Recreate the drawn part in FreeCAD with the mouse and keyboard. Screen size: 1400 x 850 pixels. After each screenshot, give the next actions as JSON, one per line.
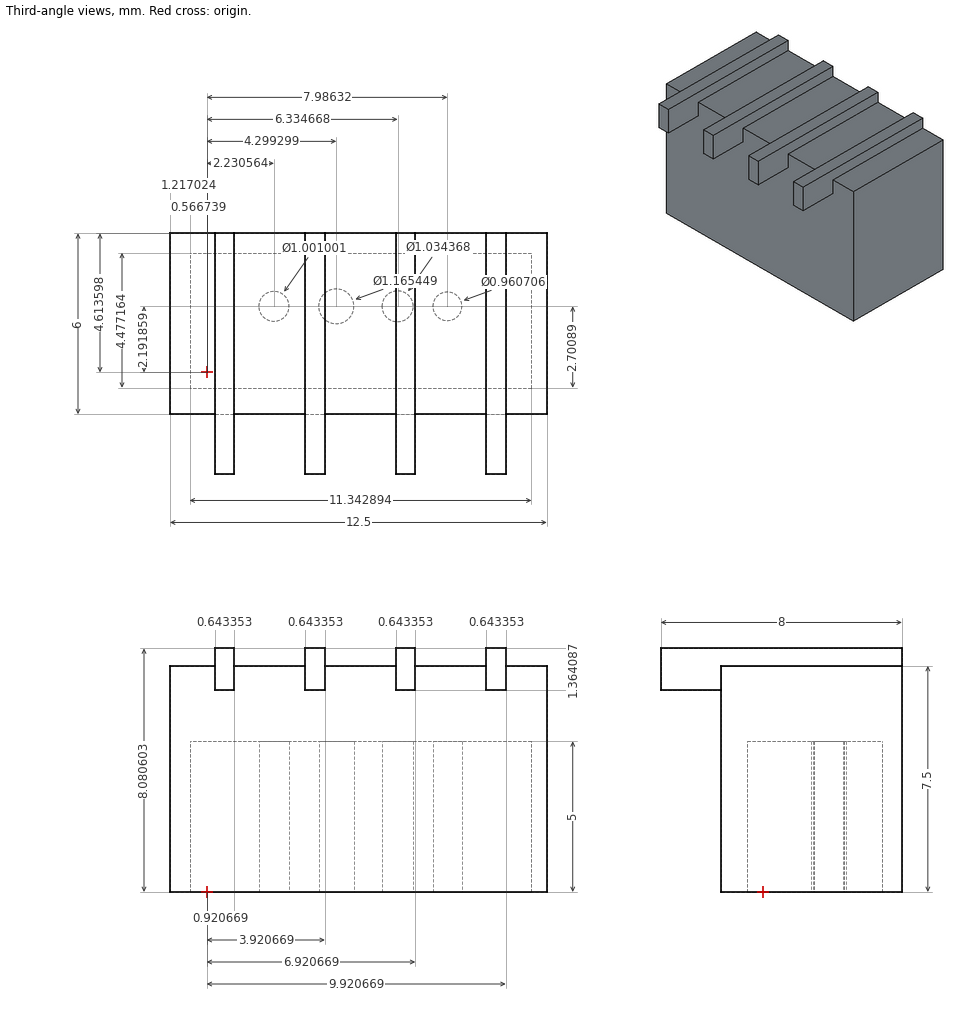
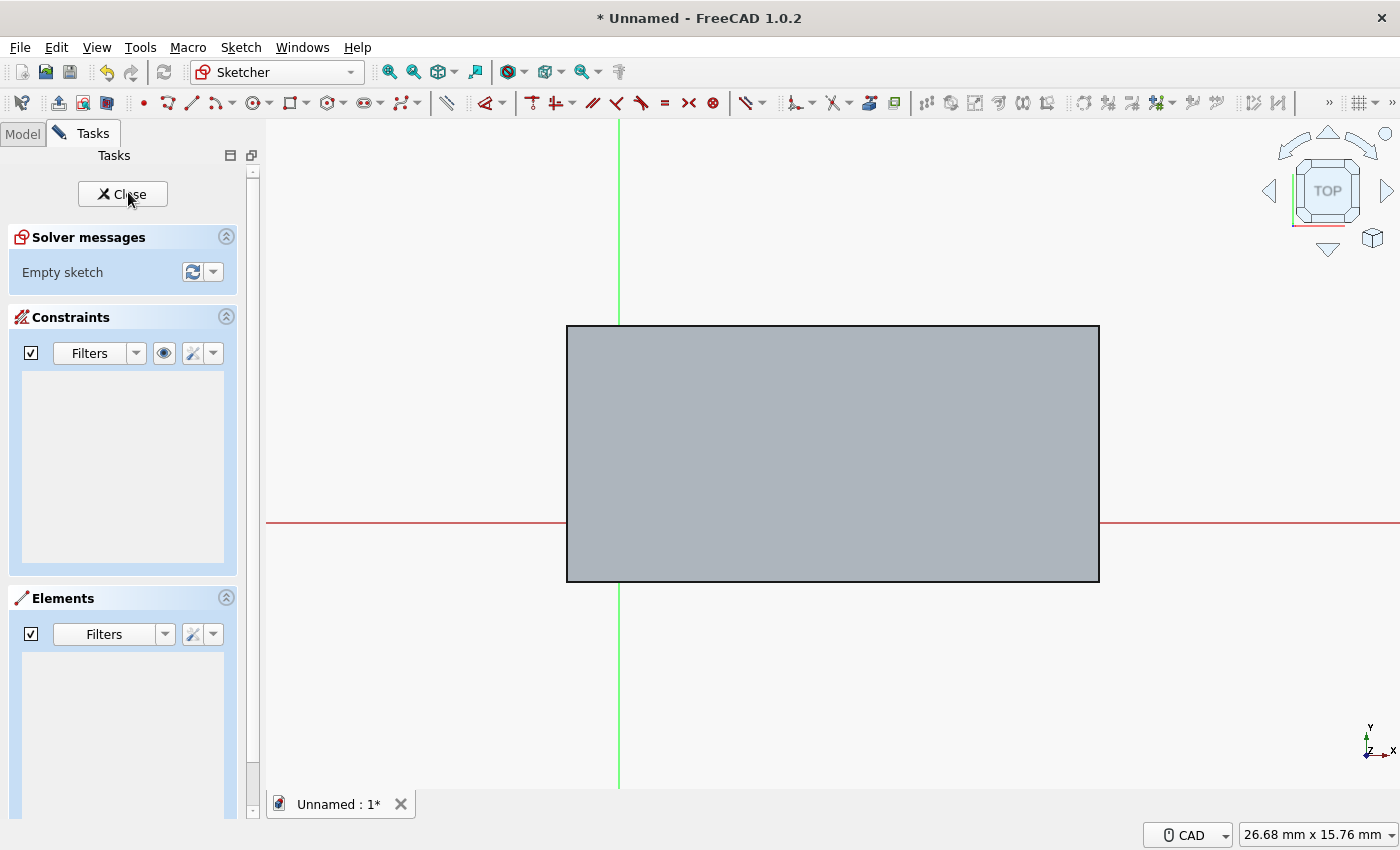
{"action": "key", "text": "q s"}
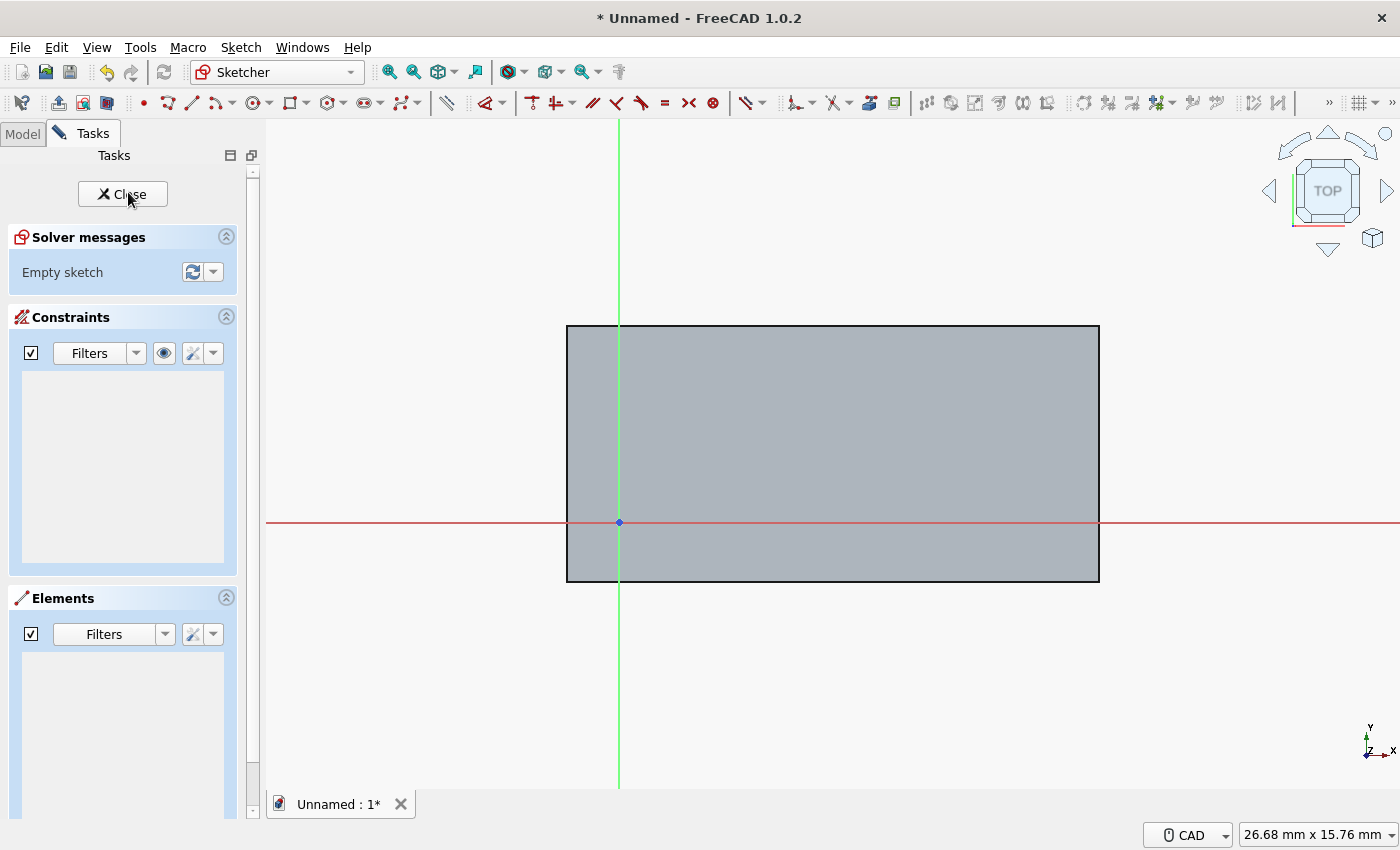
{"action": "scroll", "coordinate": [982, 439], "scroll_direction": "up", "scroll_amount": 2}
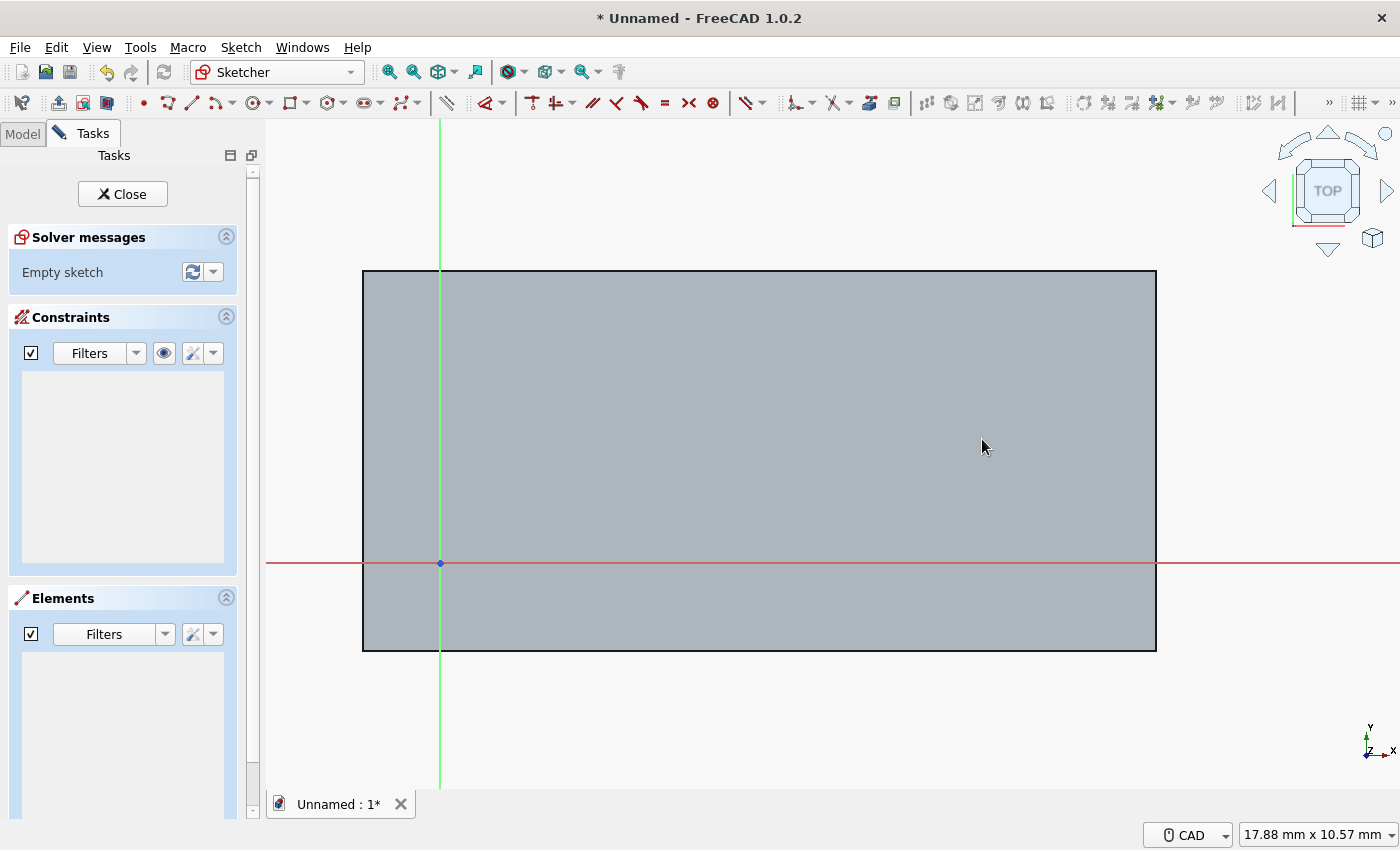
{"action": "left_click", "coordinate": [290, 104]}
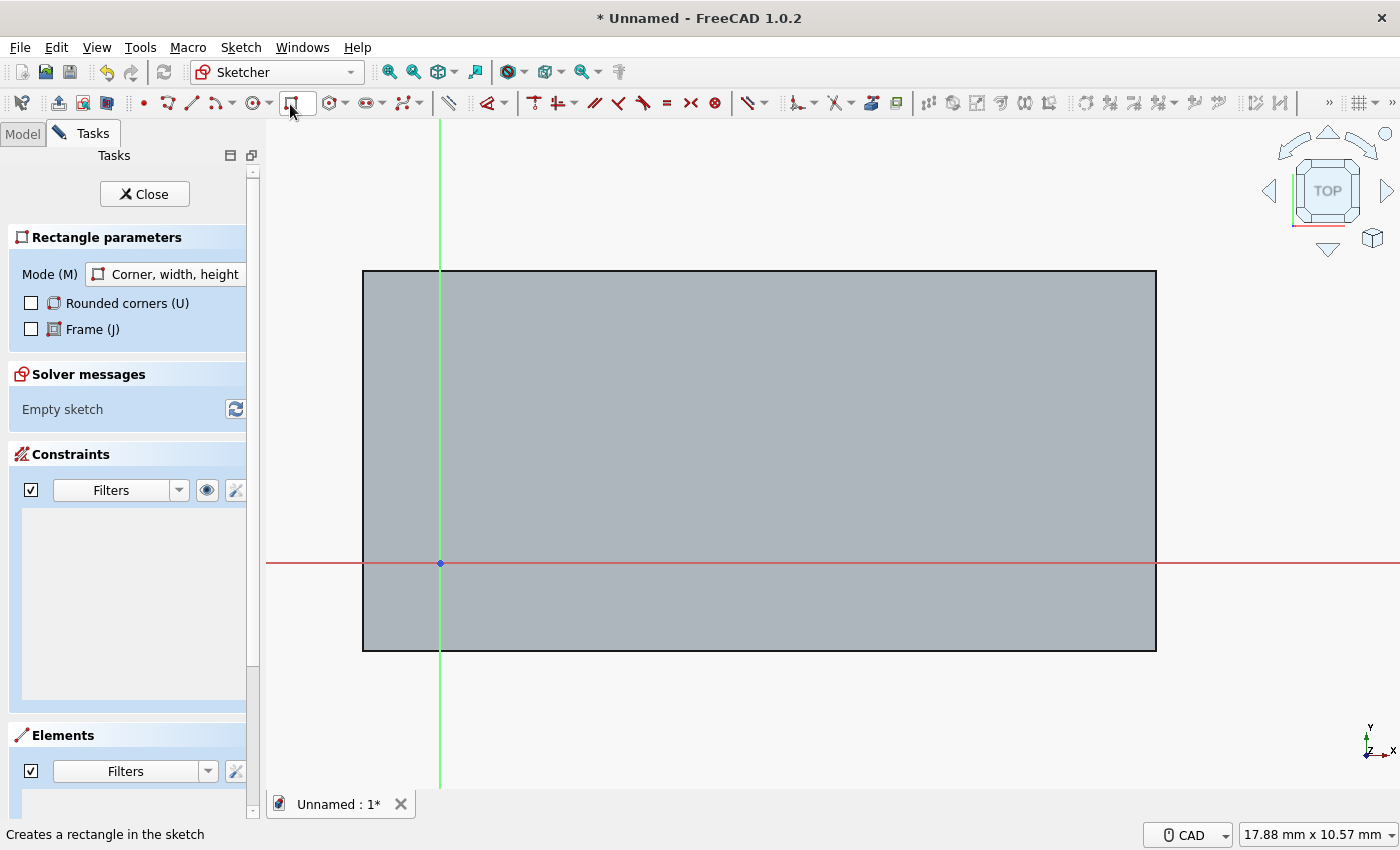
{"action": "left_click", "coordinate": [404, 312]}
{"action": "left_click", "coordinate": [1124, 596]}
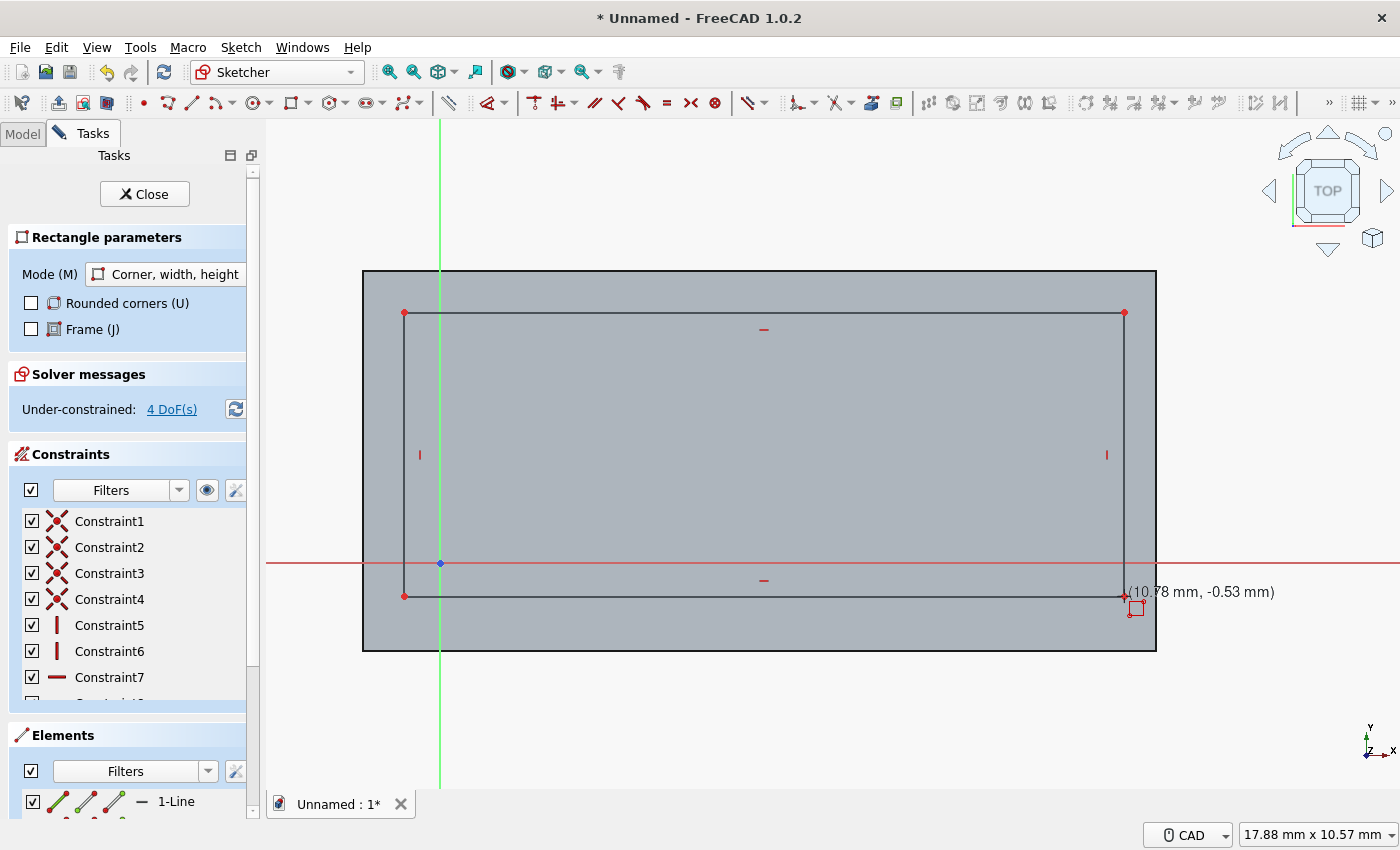
{"action": "key", "text": "g c"}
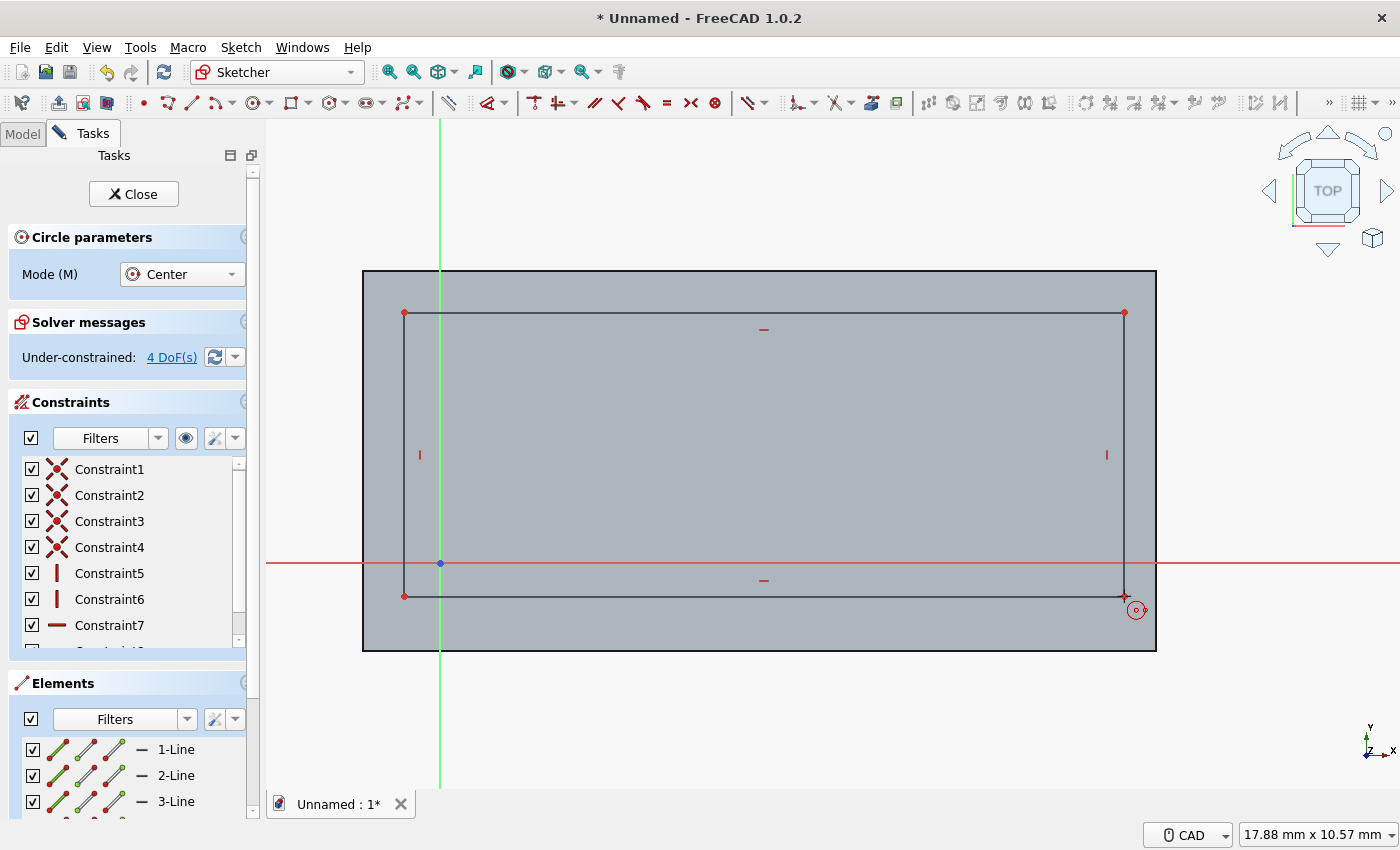
{"action": "left_click", "coordinate": [947, 424]}
{"action": "left_click", "coordinate": [968, 403]}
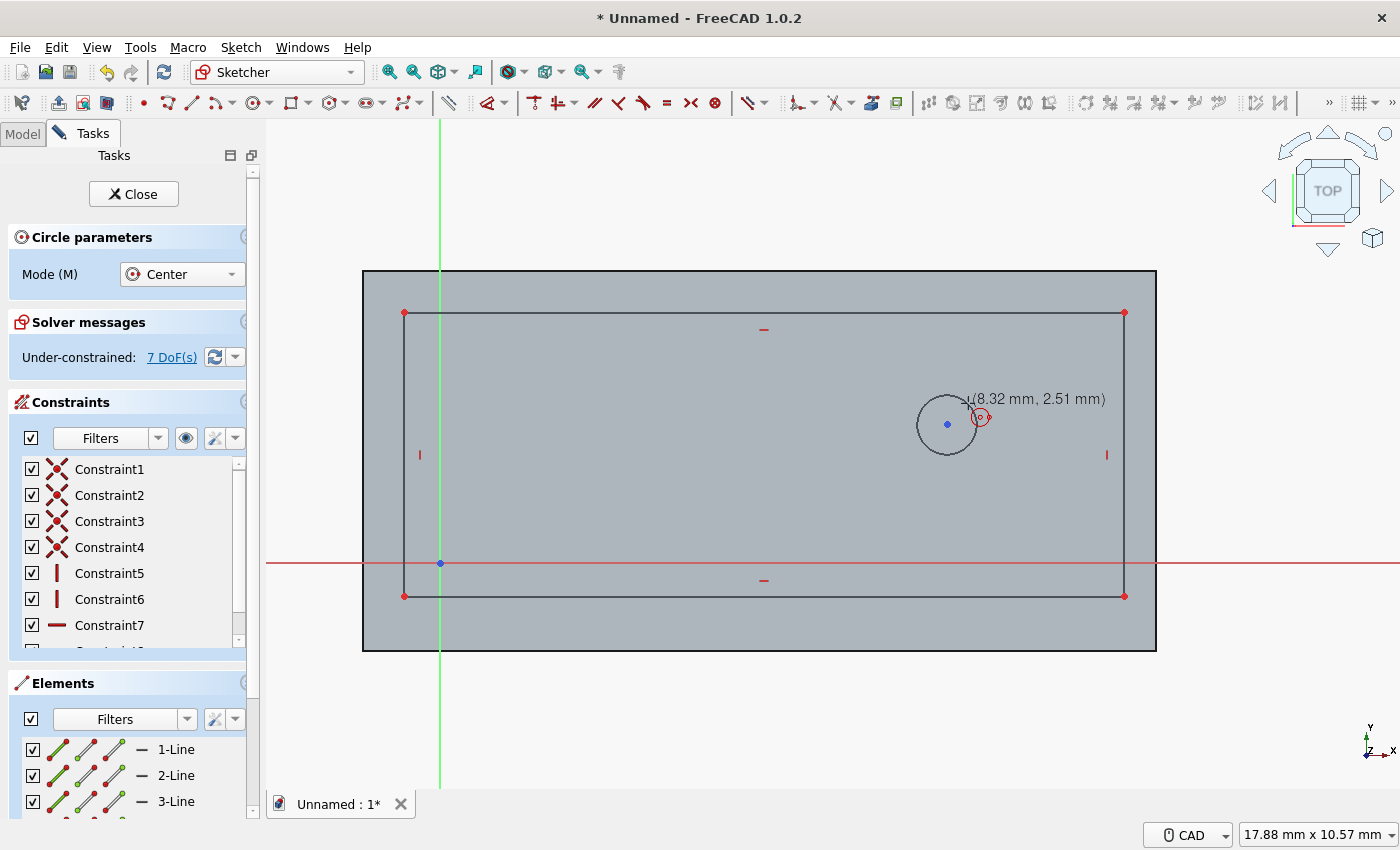
{"action": "left_click", "coordinate": [842, 424]}
{"action": "left_click", "coordinate": [865, 401]}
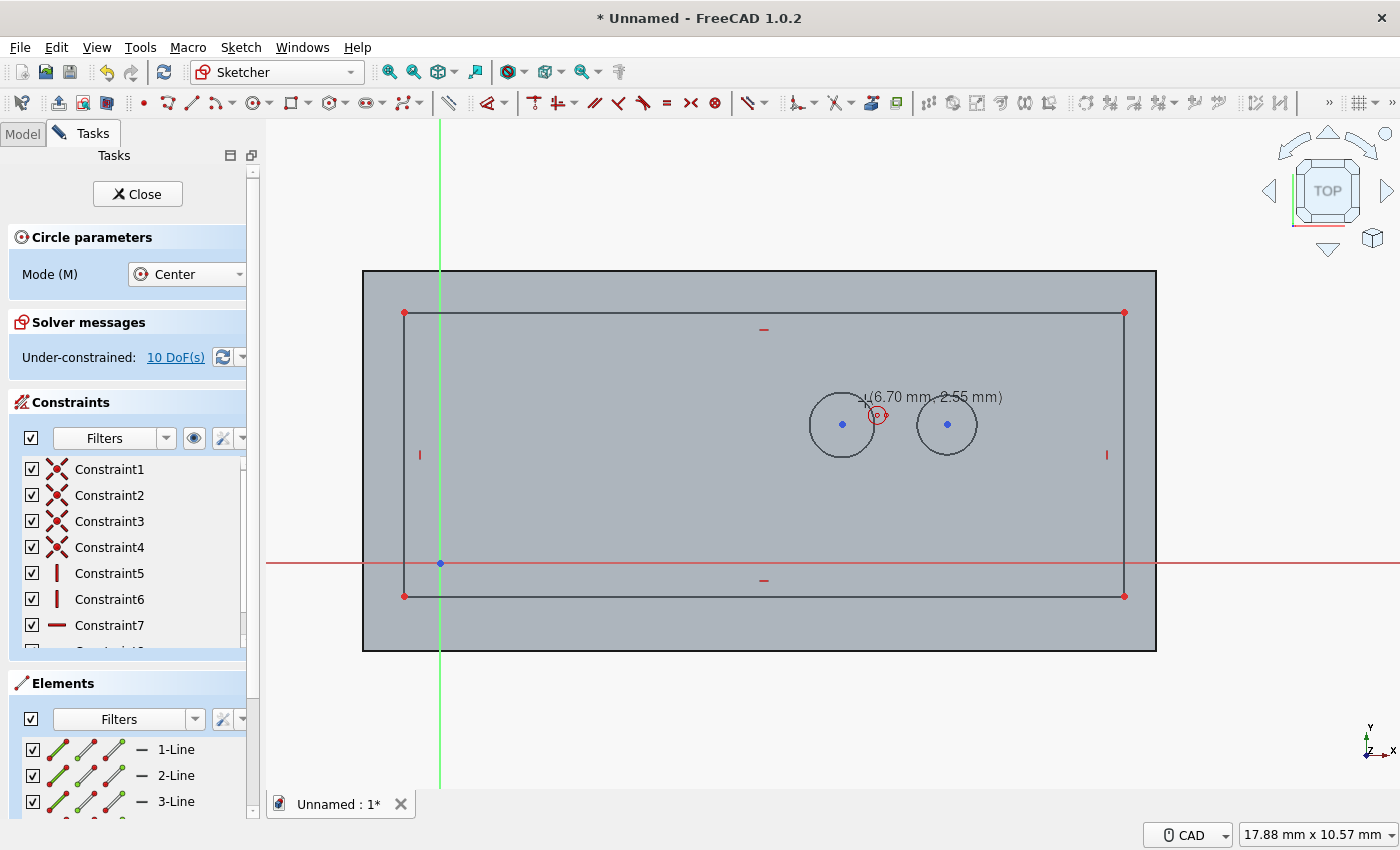
{"action": "left_click", "coordinate": [713, 424]}
{"action": "left_click", "coordinate": [739, 398]}